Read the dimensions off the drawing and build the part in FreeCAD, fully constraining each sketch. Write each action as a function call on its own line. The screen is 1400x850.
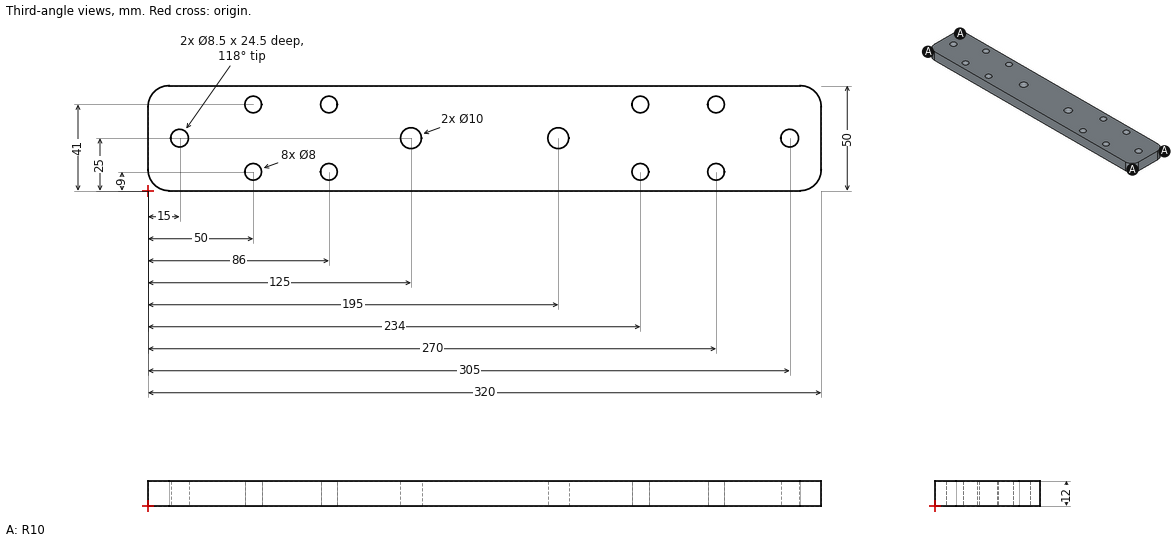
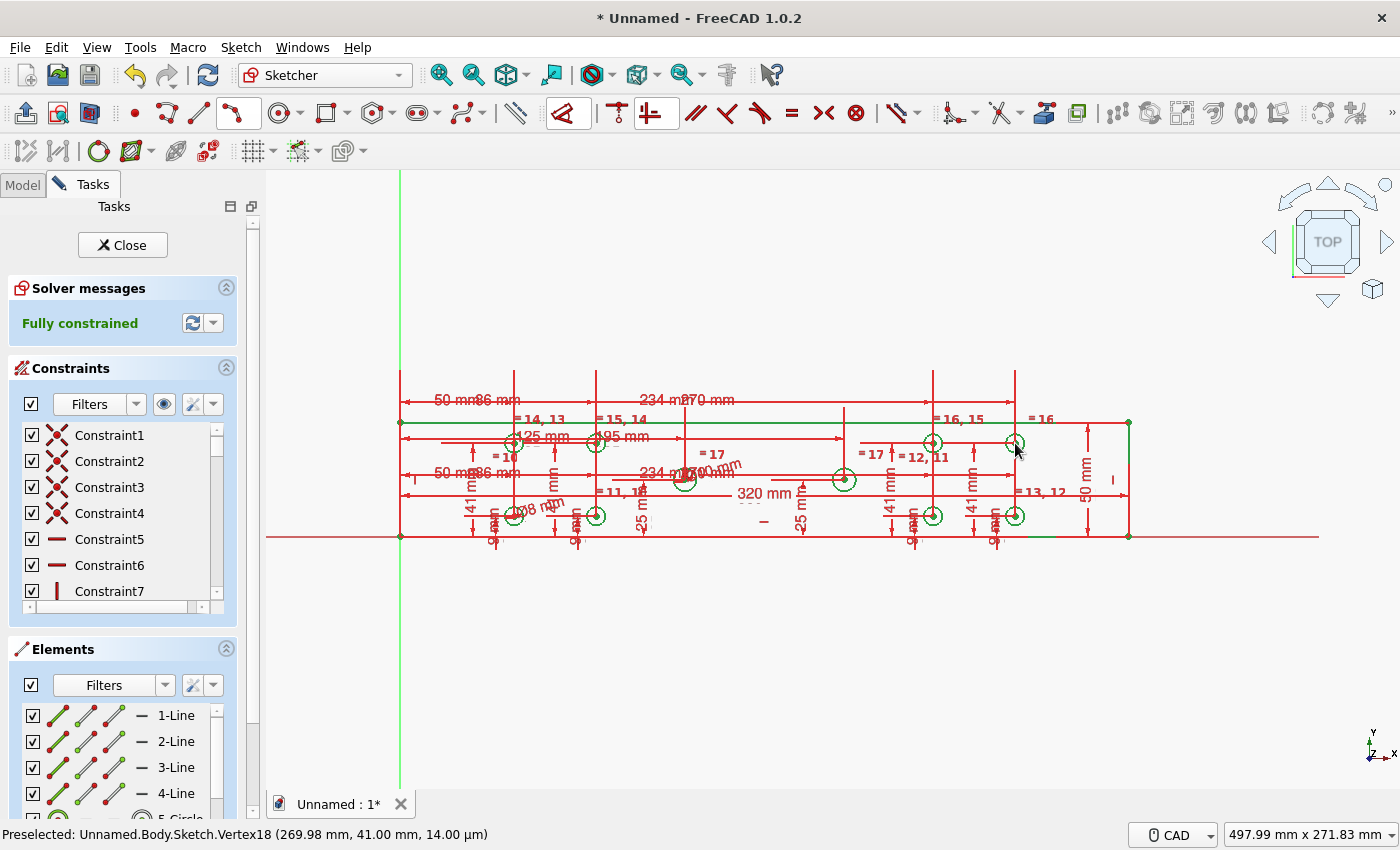
click(123, 245)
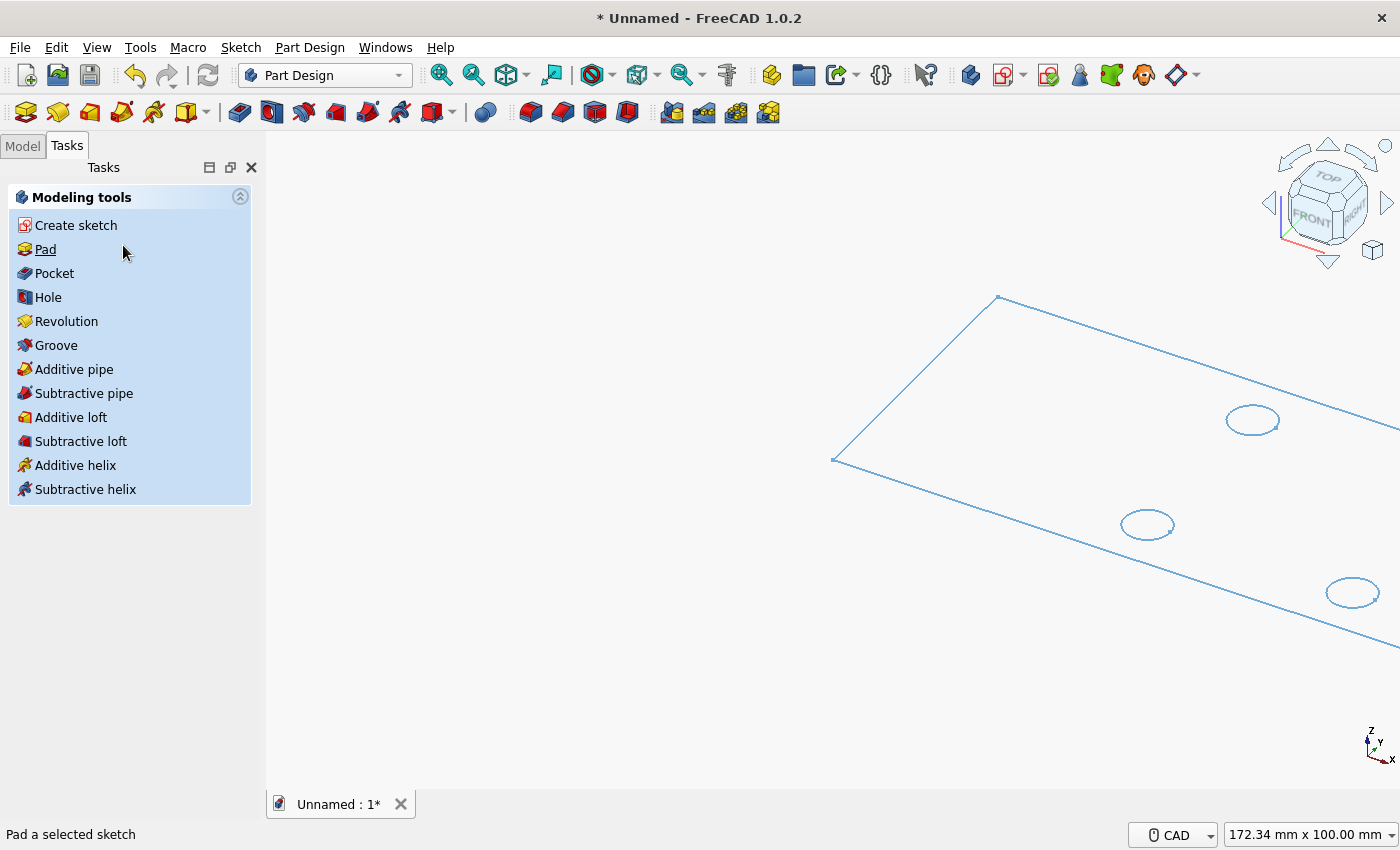
click(26, 112)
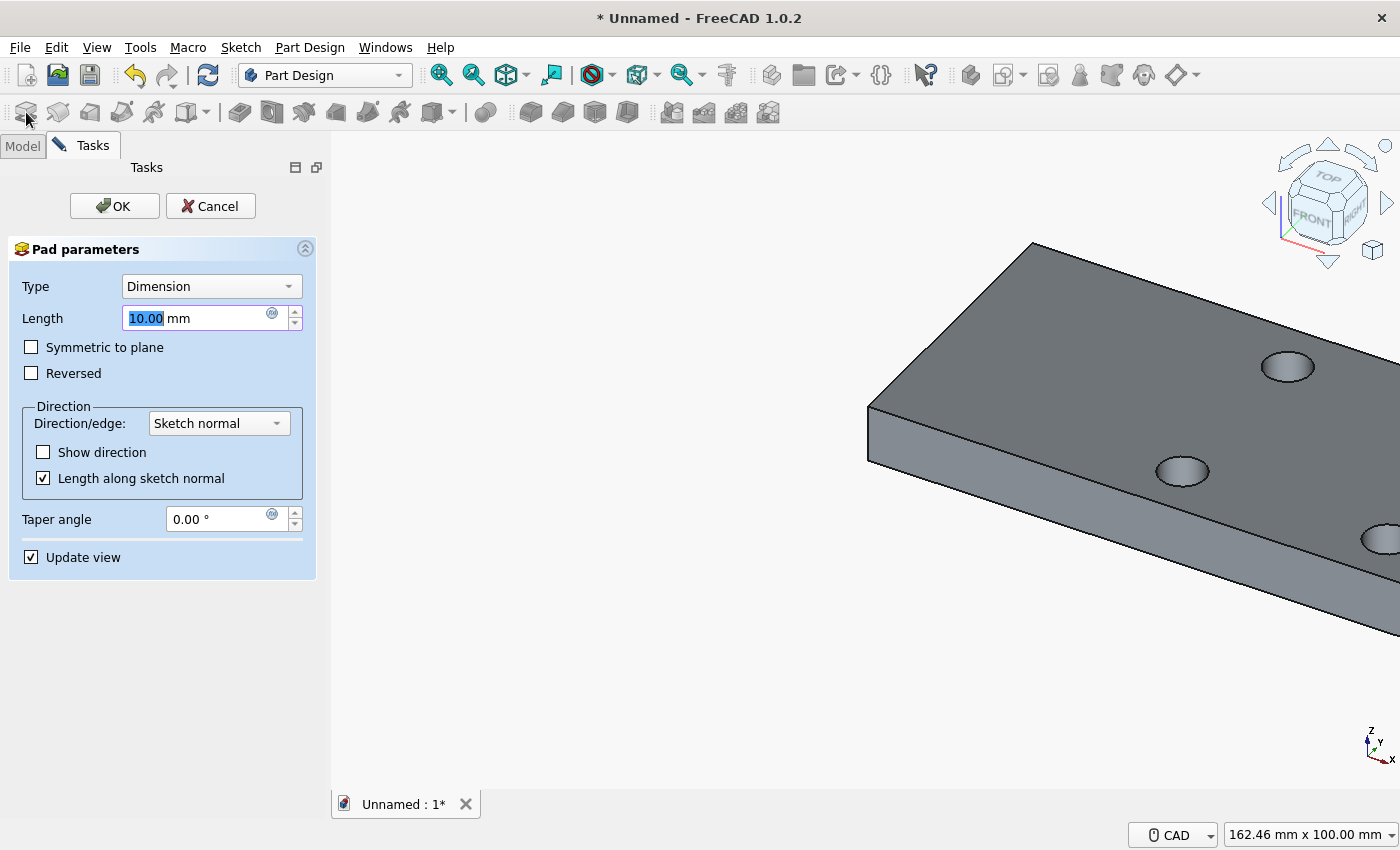
text(12)
key(Tab)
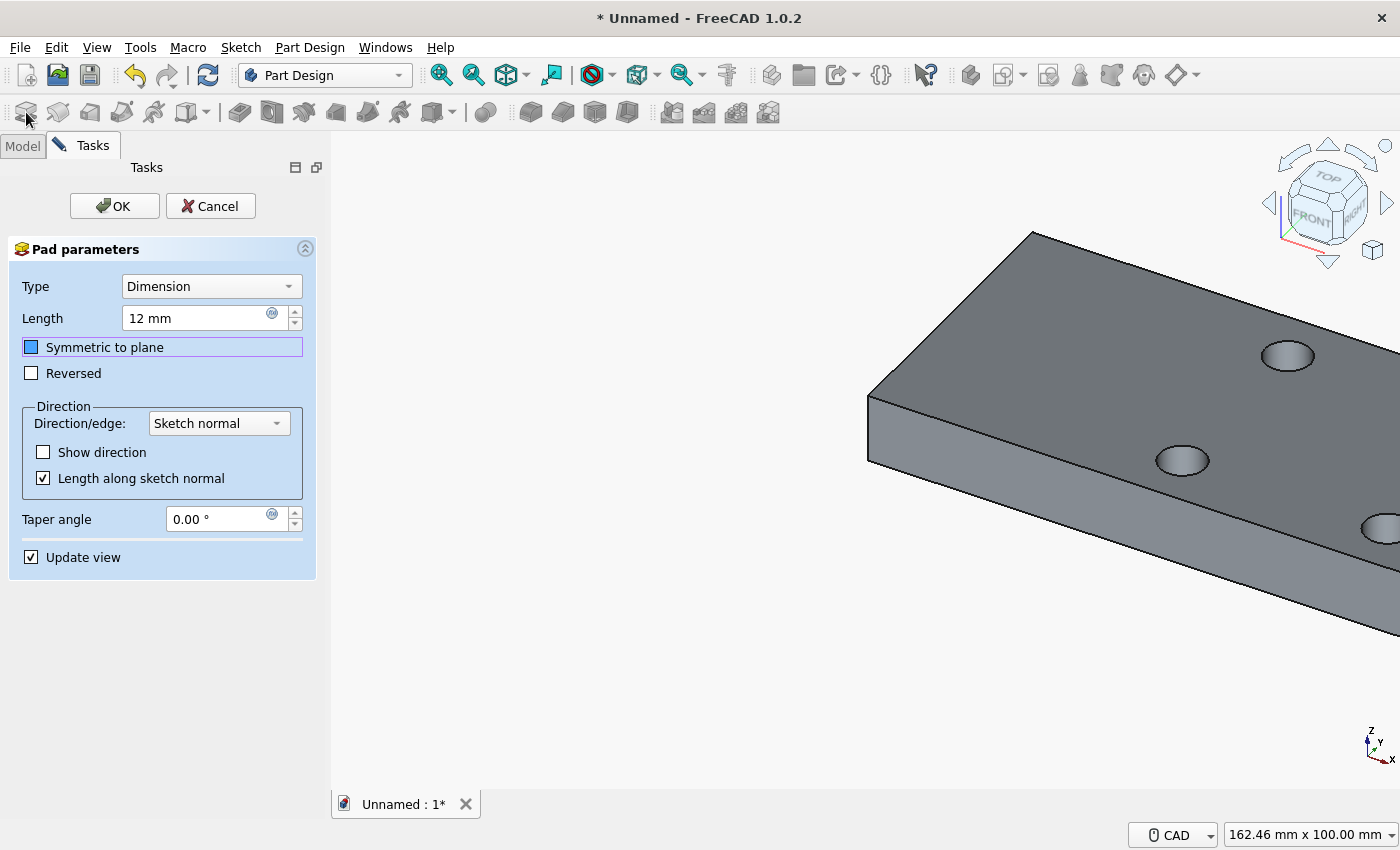
click(115, 206)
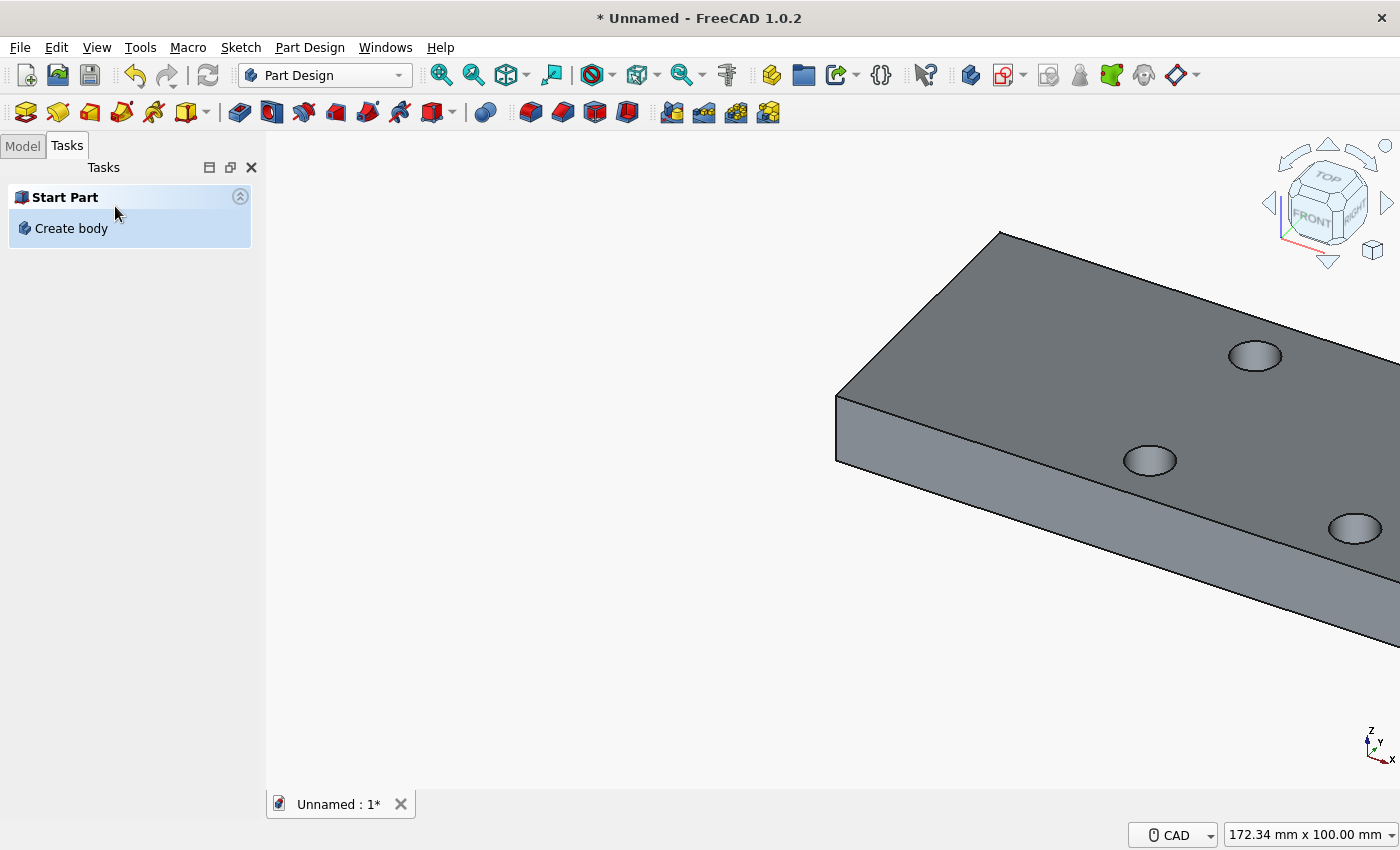
click(442, 76)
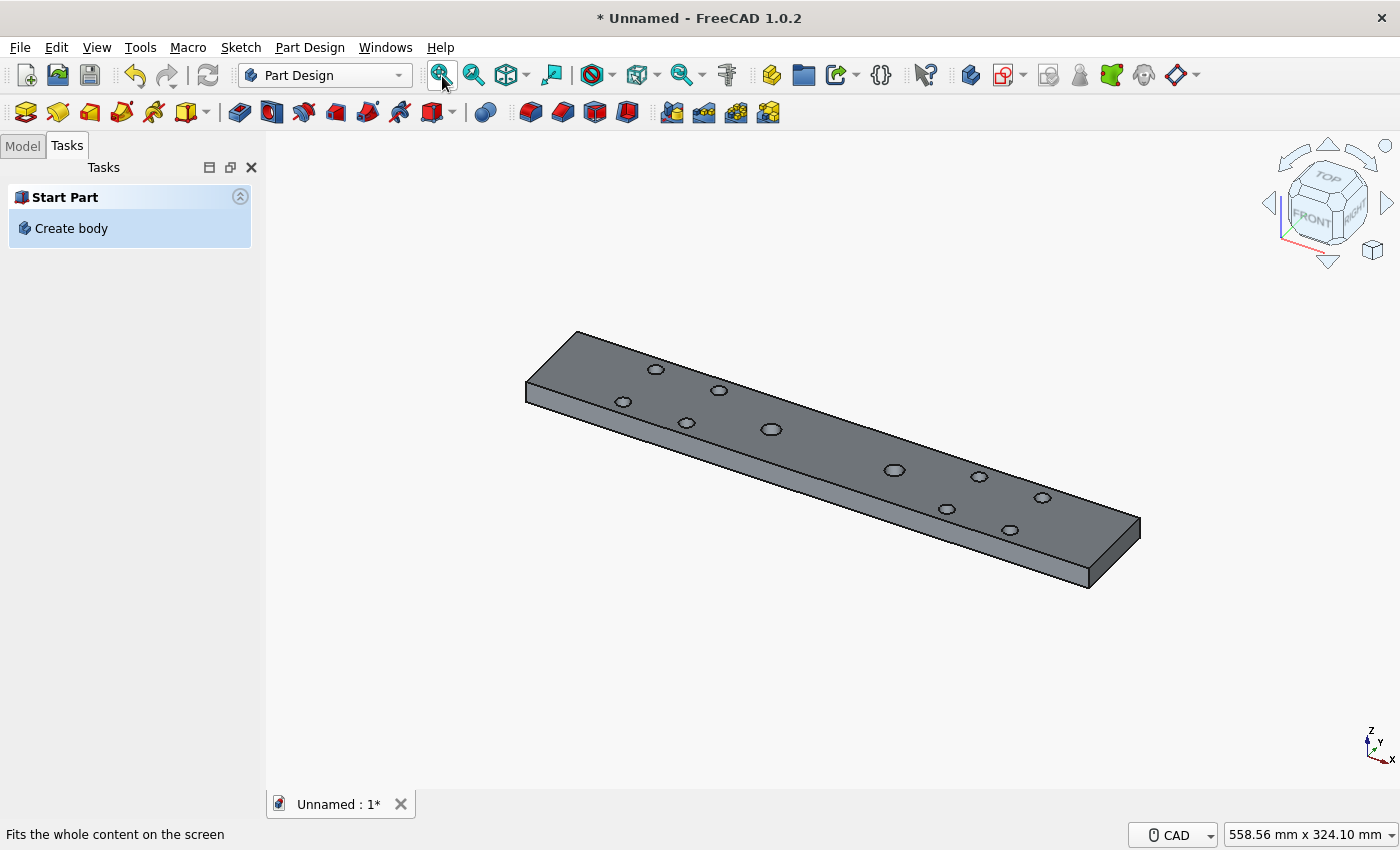
click(833, 449)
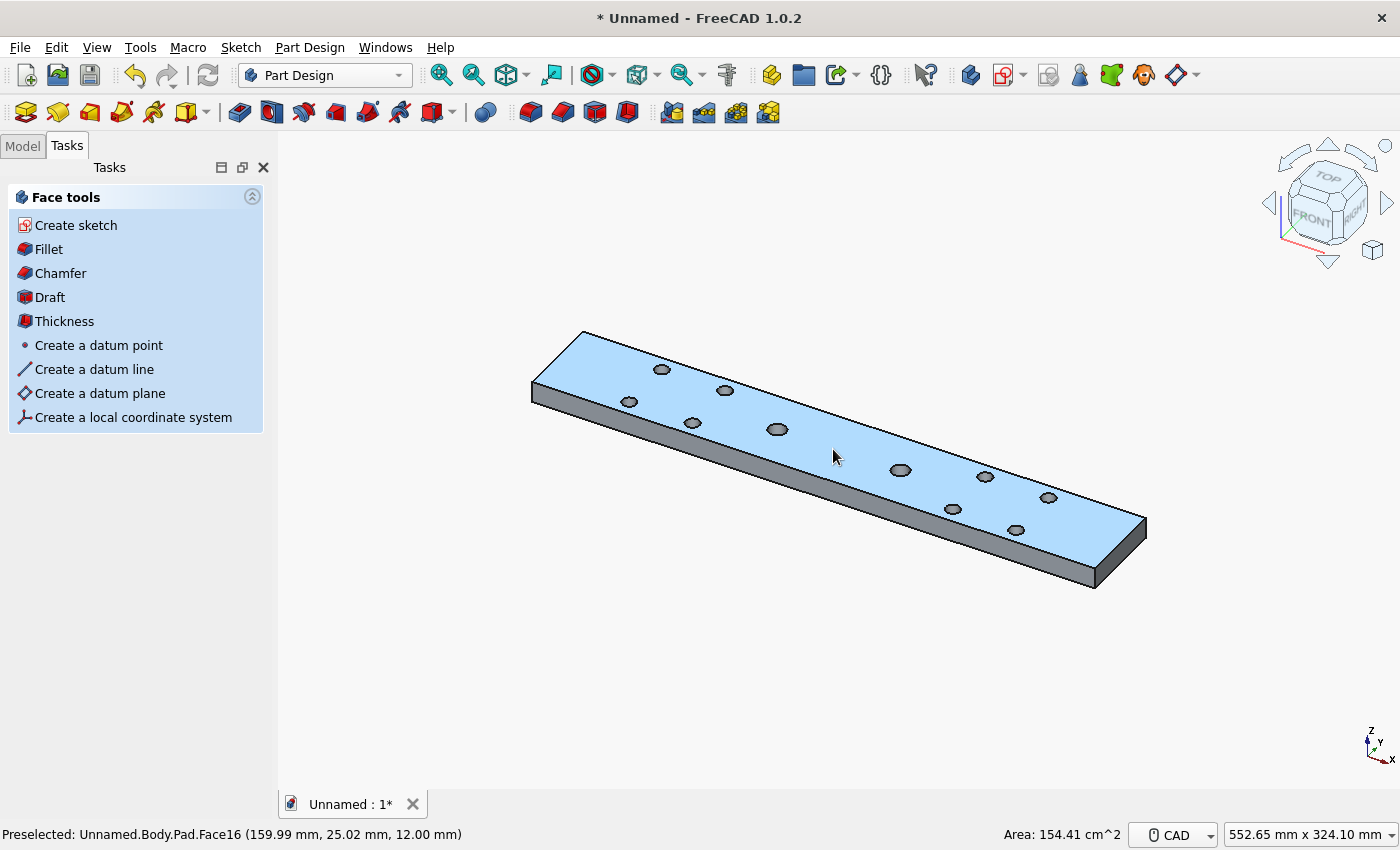
click(1004, 76)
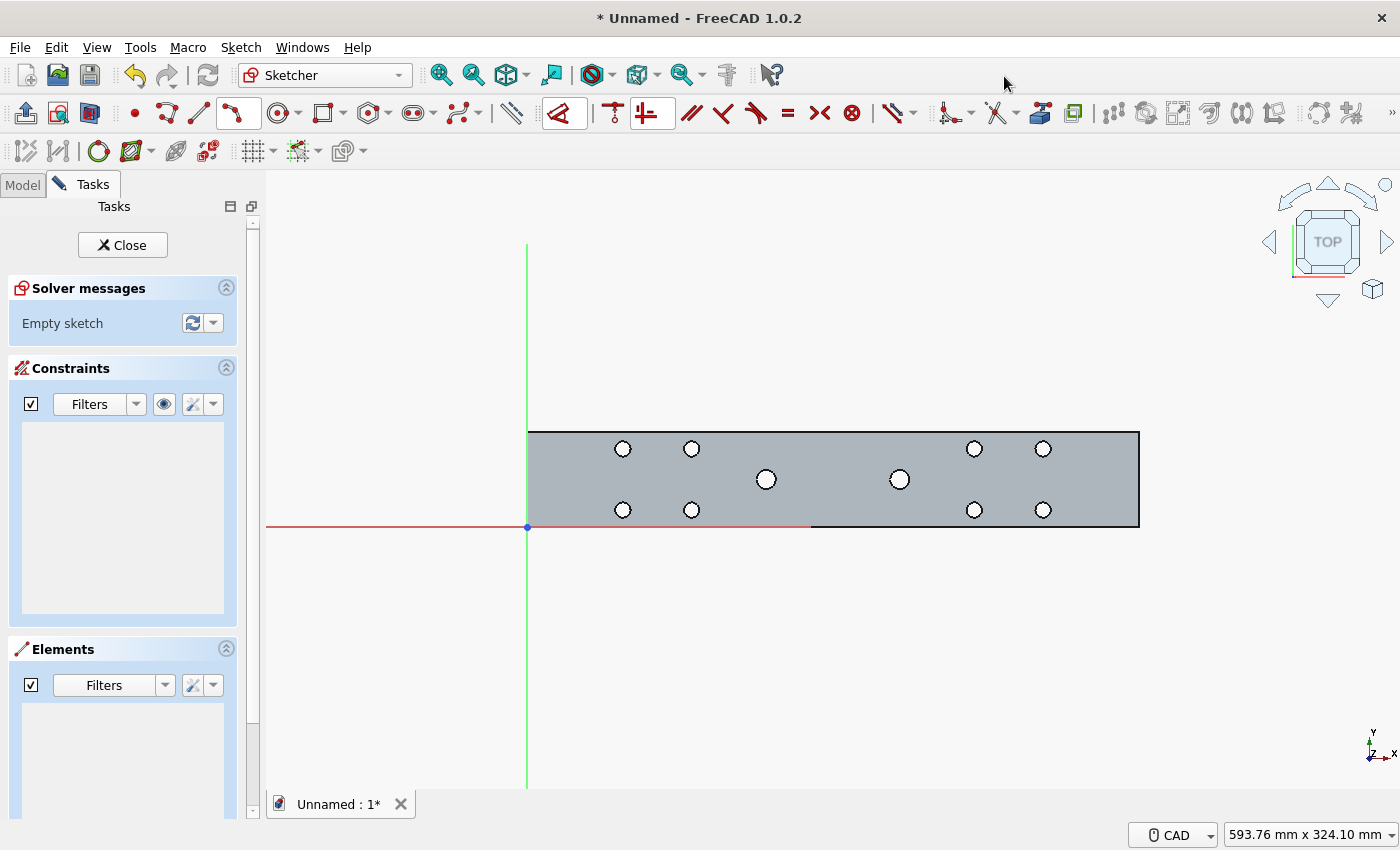
click(278, 114)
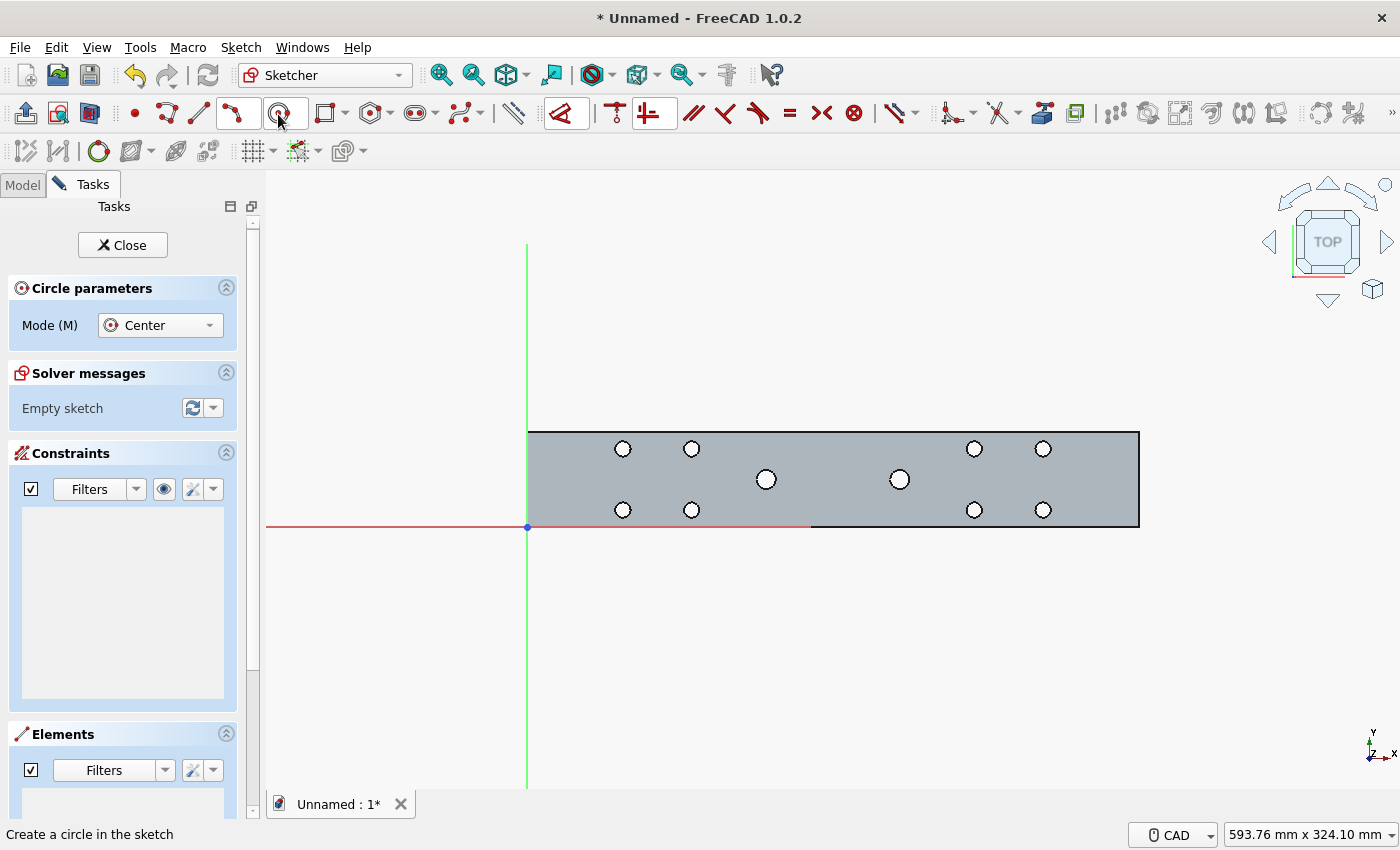
scroll(556, 480, up, 6)